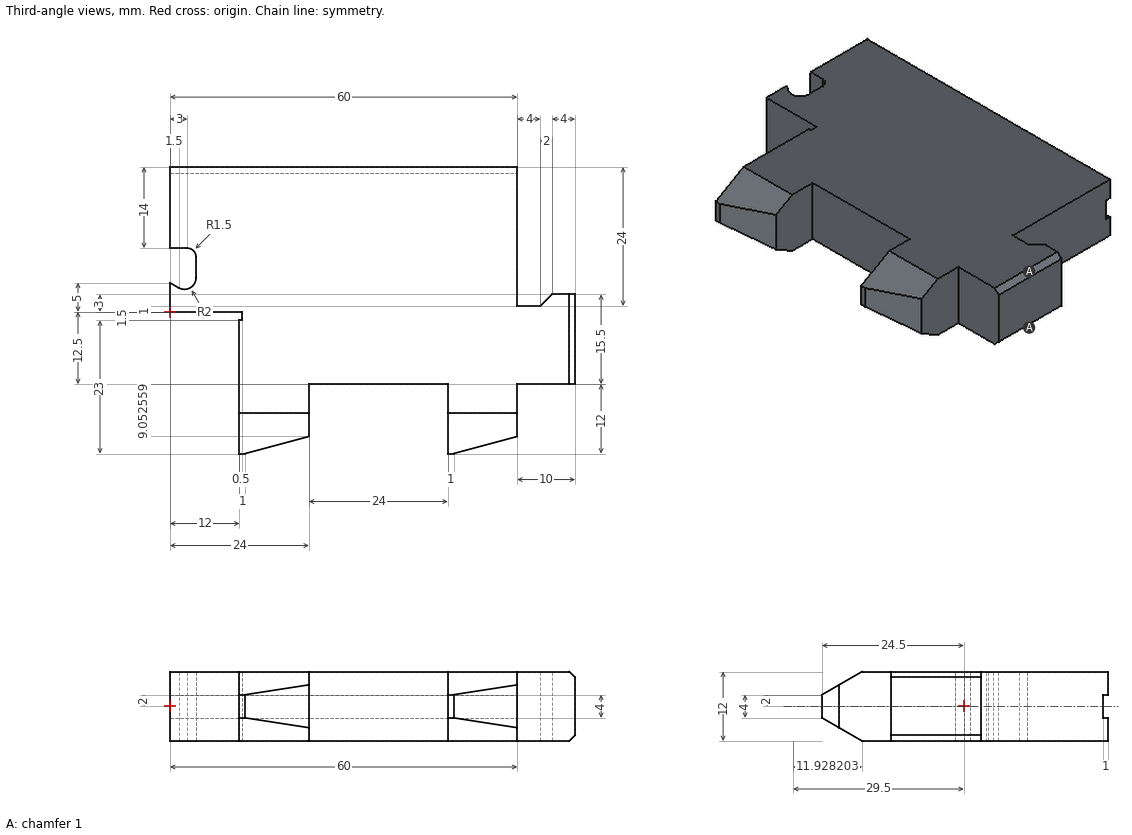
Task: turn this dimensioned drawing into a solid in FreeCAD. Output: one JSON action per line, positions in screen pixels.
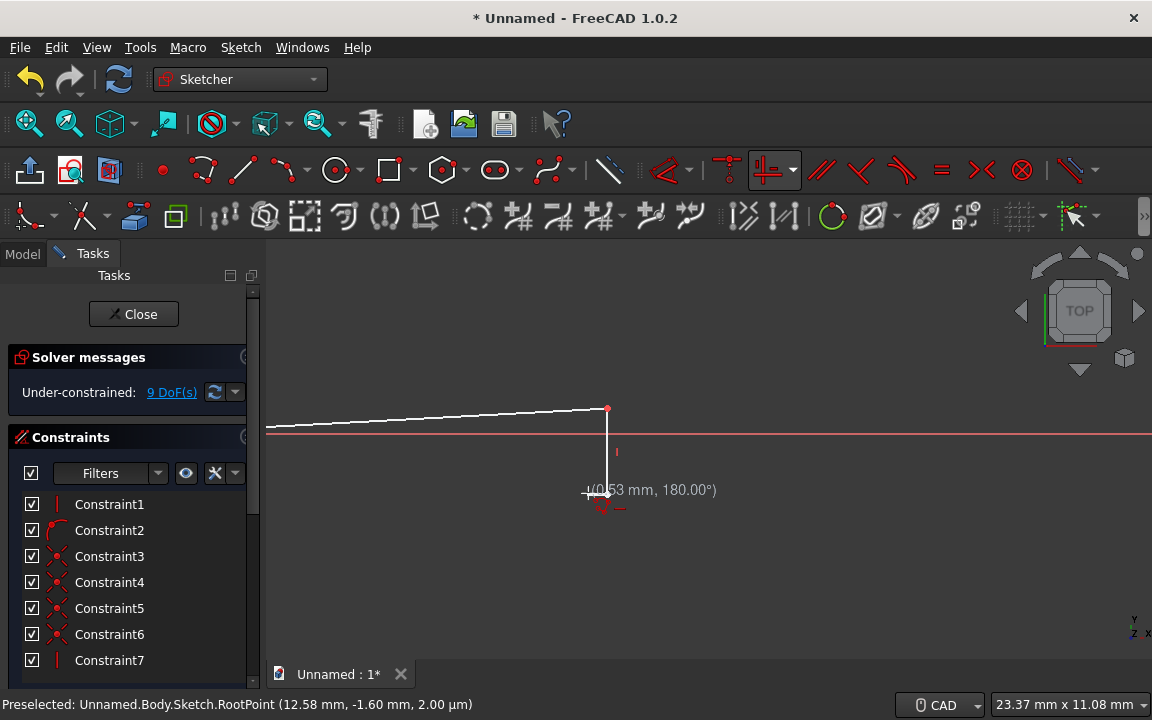
{"action": "left_click", "coordinate": [588, 492]}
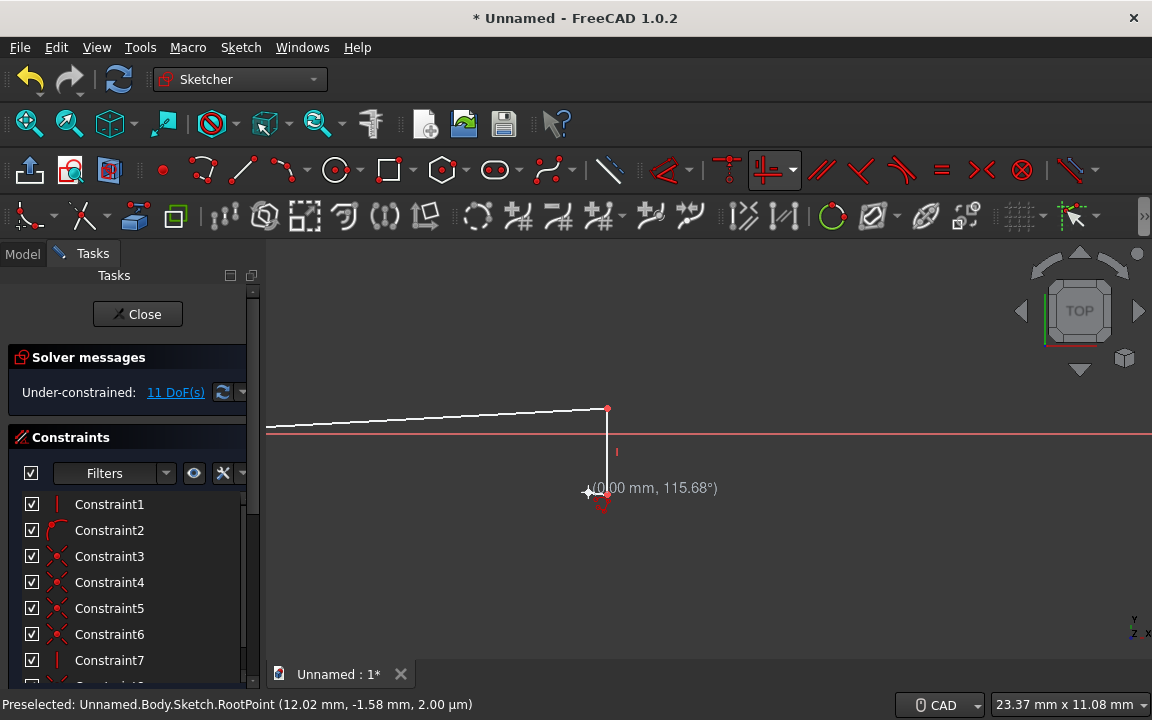
{"action": "scroll", "coordinate": [512, 453], "scroll_direction": "down", "scroll_amount": 10}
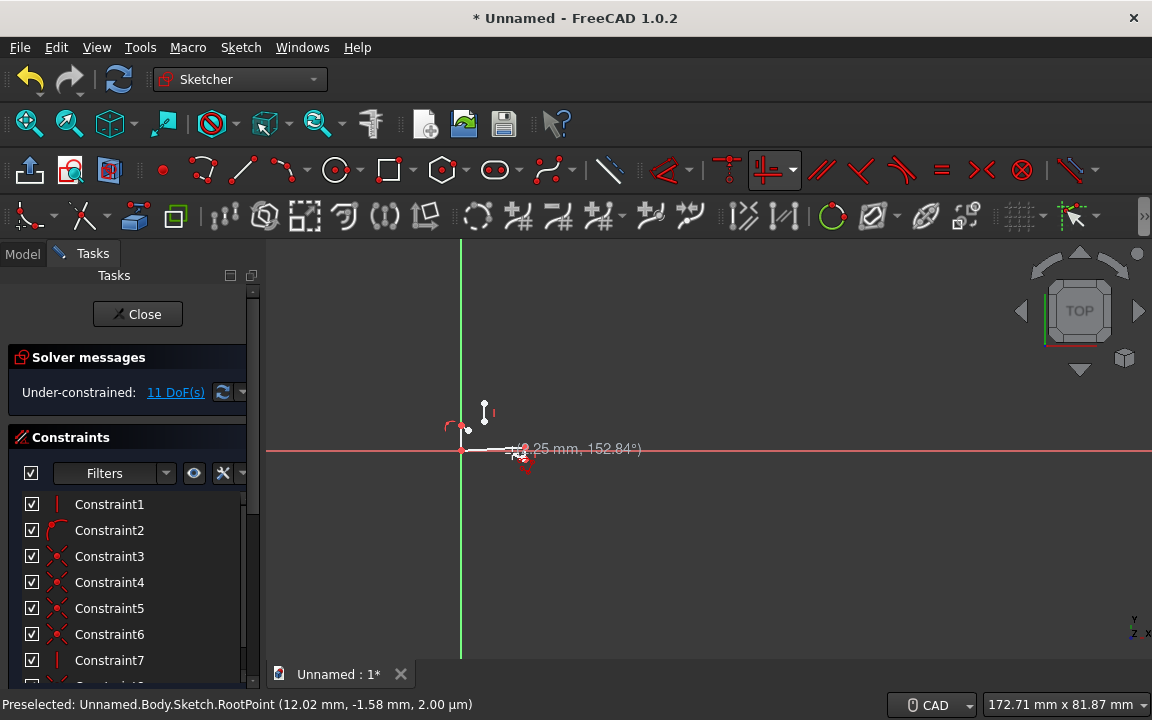
{"action": "left_click", "coordinate": [523, 577]}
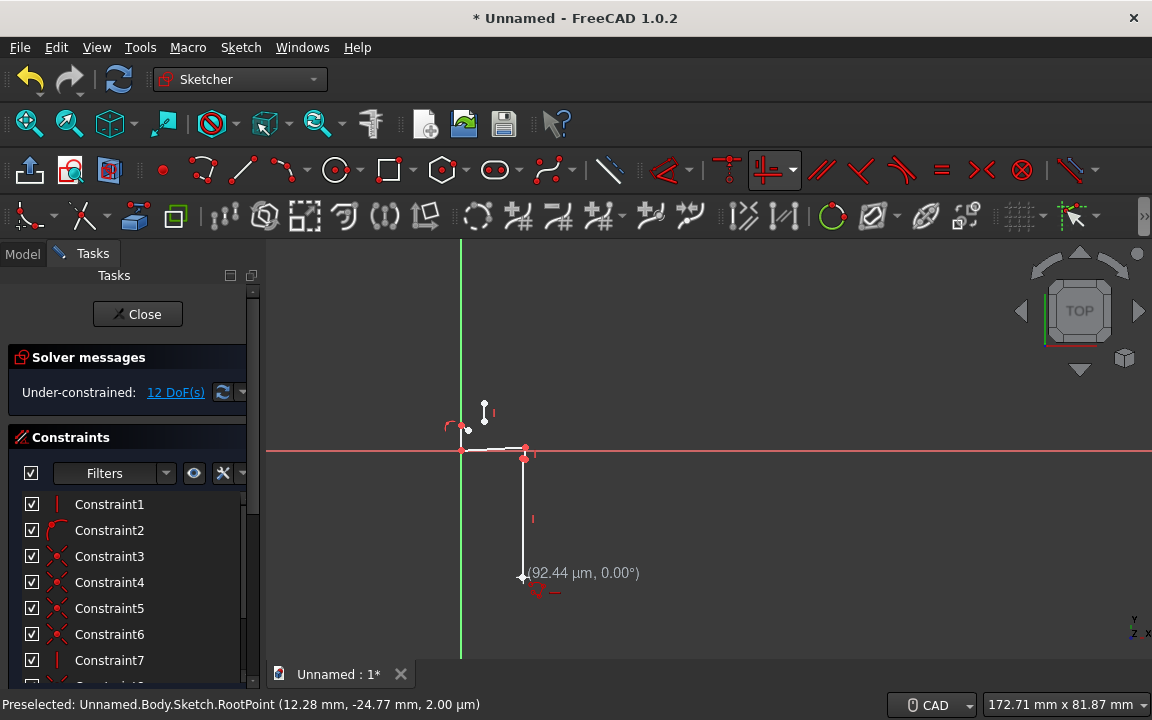
{"action": "scroll", "coordinate": [528, 577], "scroll_direction": "up", "scroll_amount": 6}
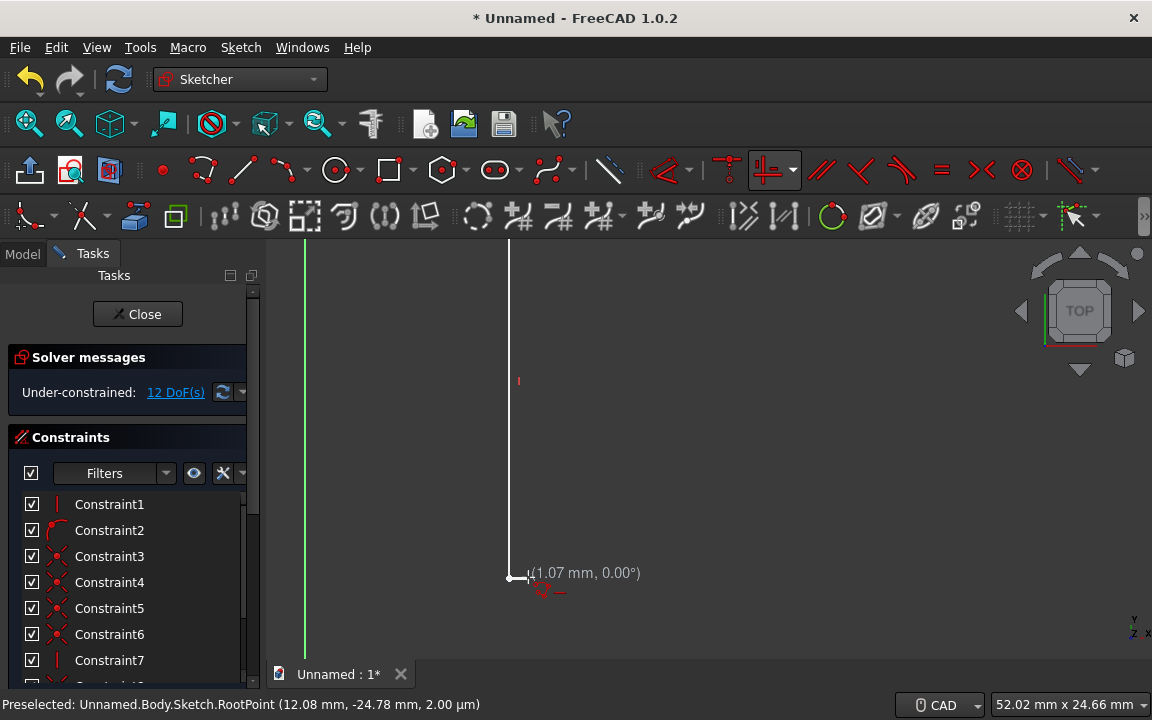
{"action": "left_click", "coordinate": [526, 575]}
{"action": "left_click", "coordinate": [714, 524]}
{"action": "left_click", "coordinate": [714, 369]}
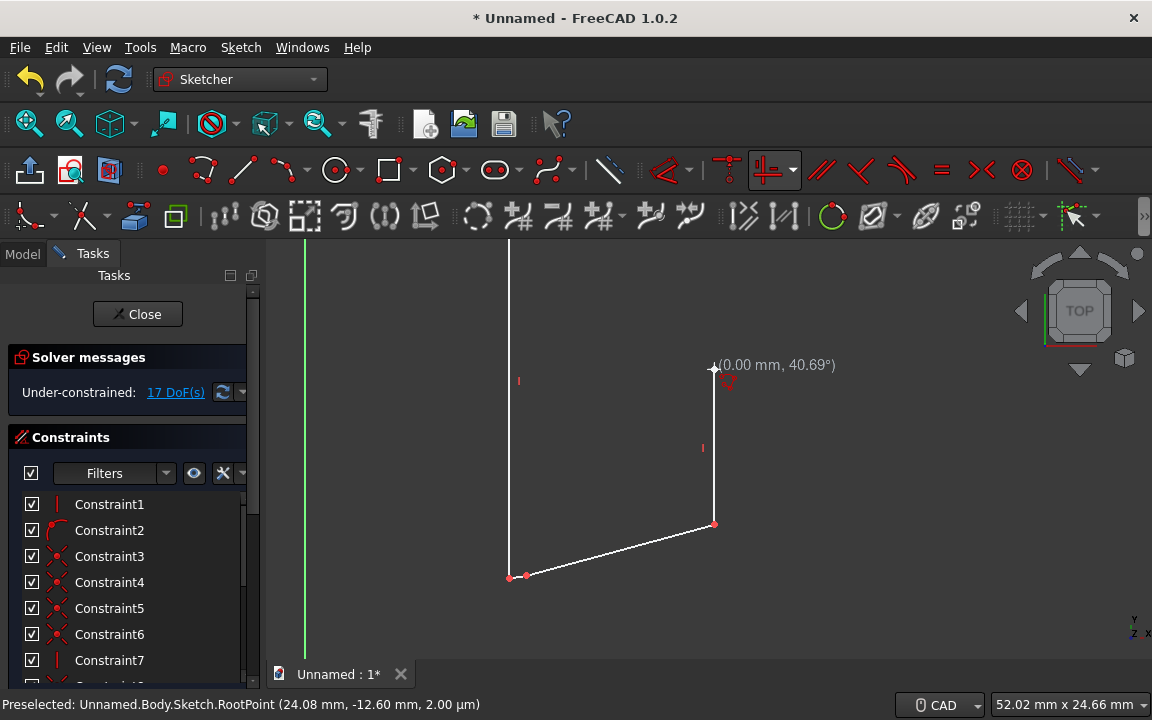
{"action": "scroll", "coordinate": [528, 577], "scroll_direction": "down", "scroll_amount": 6}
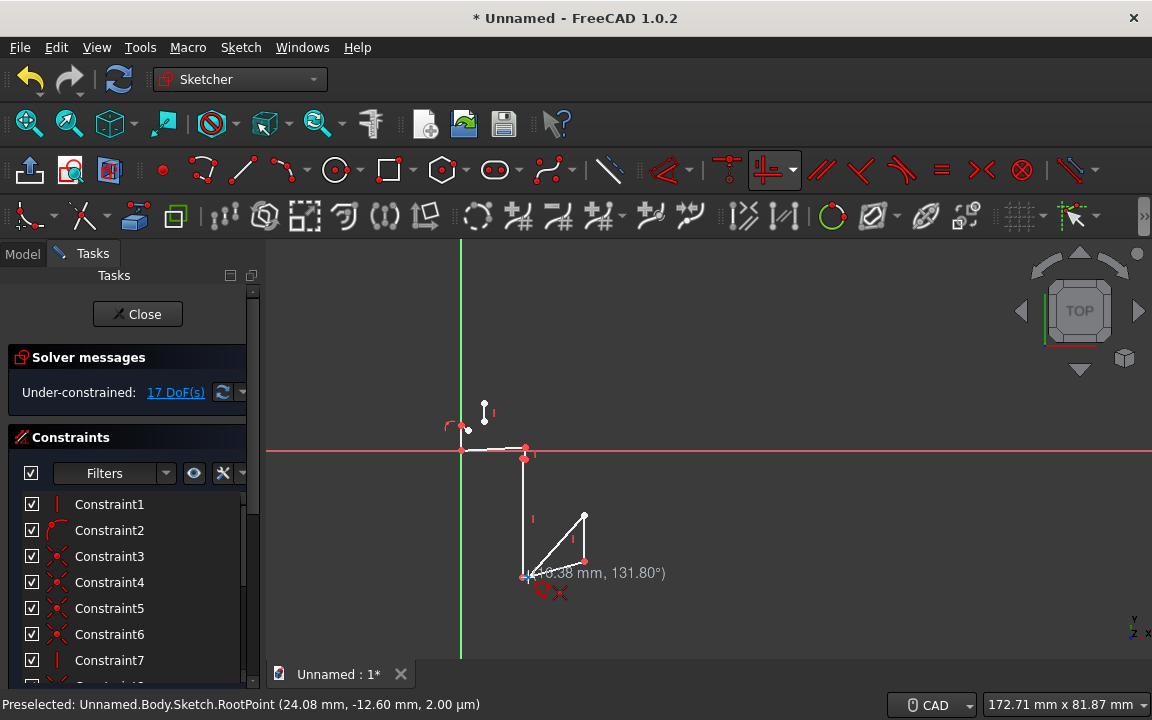
{"action": "left_click", "coordinate": [707, 515]}
{"action": "left_click", "coordinate": [707, 577]}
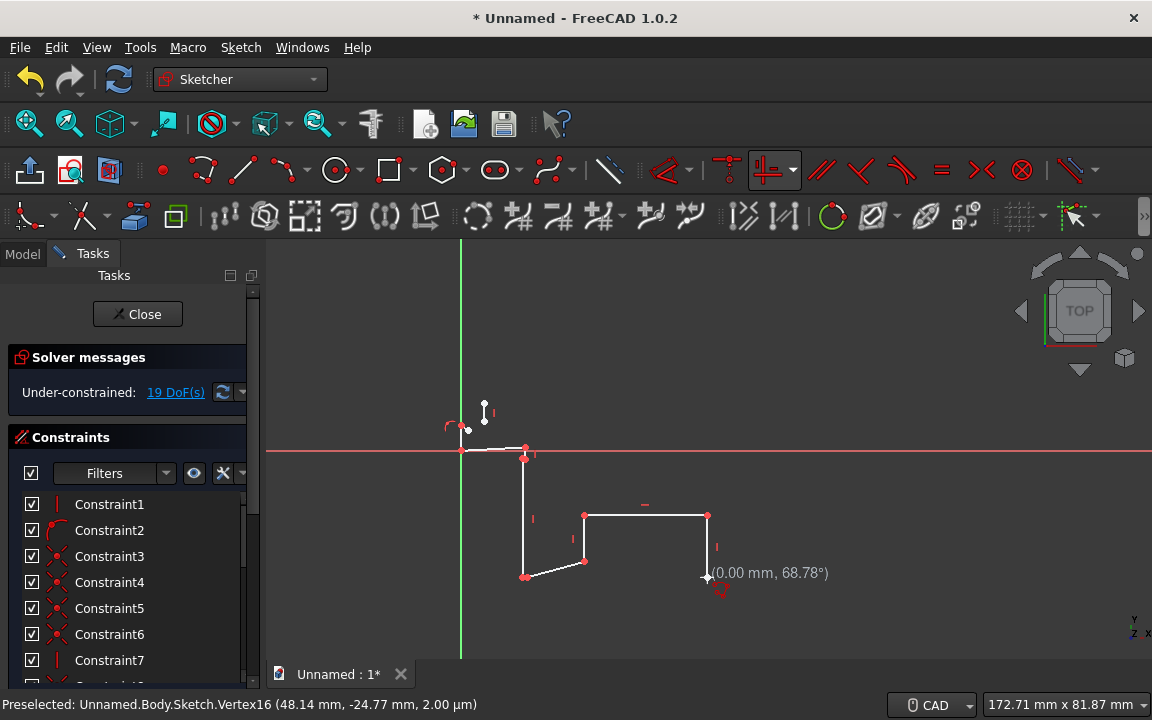
{"action": "scroll", "coordinate": [712, 577], "scroll_direction": "up", "scroll_amount": 6}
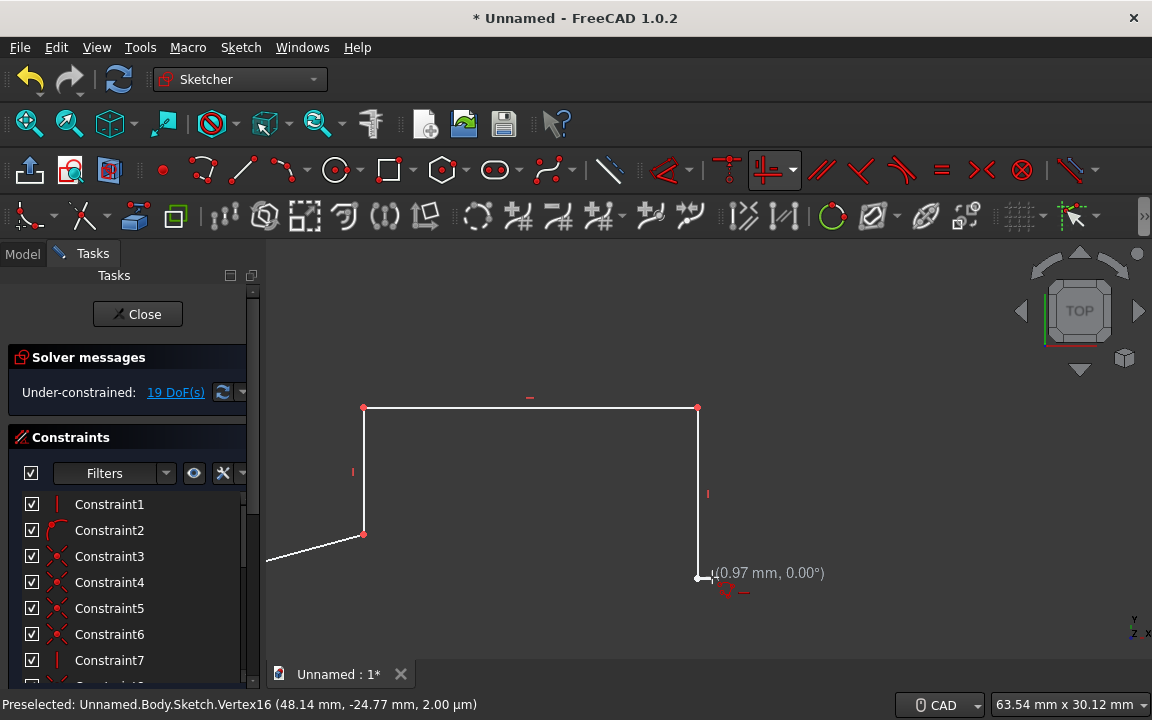
{"action": "left_click", "coordinate": [712, 575]}
{"action": "left_click", "coordinate": [899, 524]}
{"action": "left_click", "coordinate": [899, 369]}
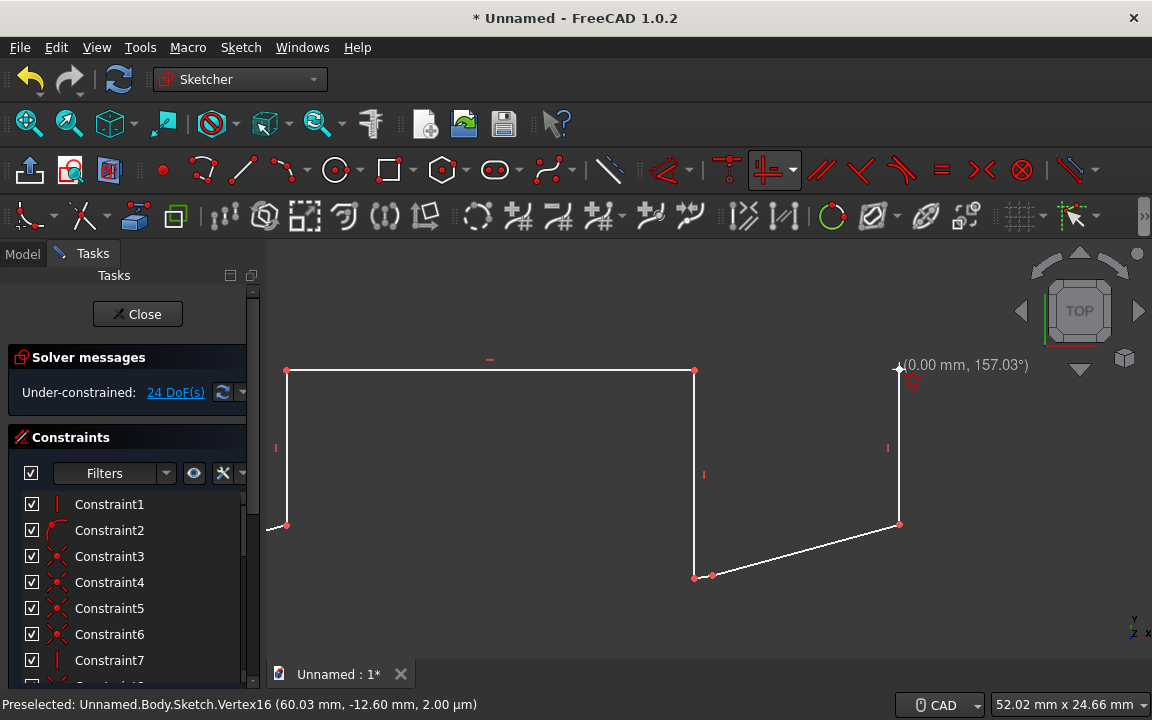
{"action": "scroll", "coordinate": [712, 577], "scroll_direction": "down", "scroll_amount": 6}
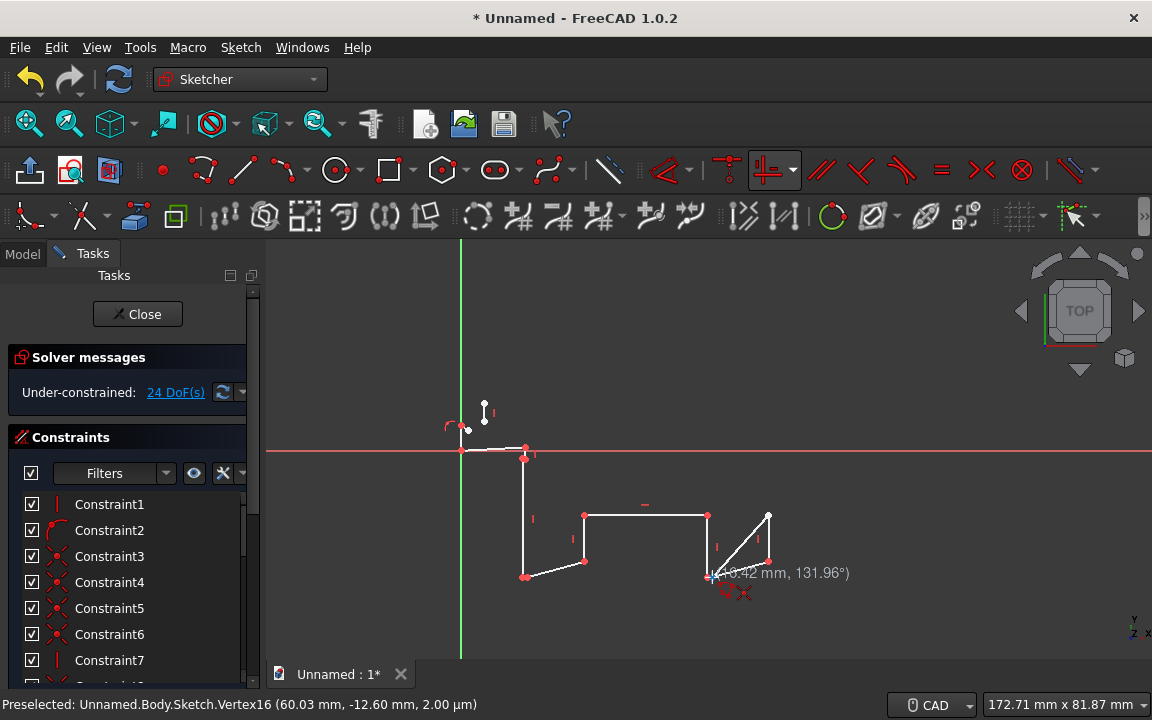
{"action": "left_click", "coordinate": [820, 515]}
{"action": "left_click", "coordinate": [820, 436]}
{"action": "left_click", "coordinate": [800, 436]}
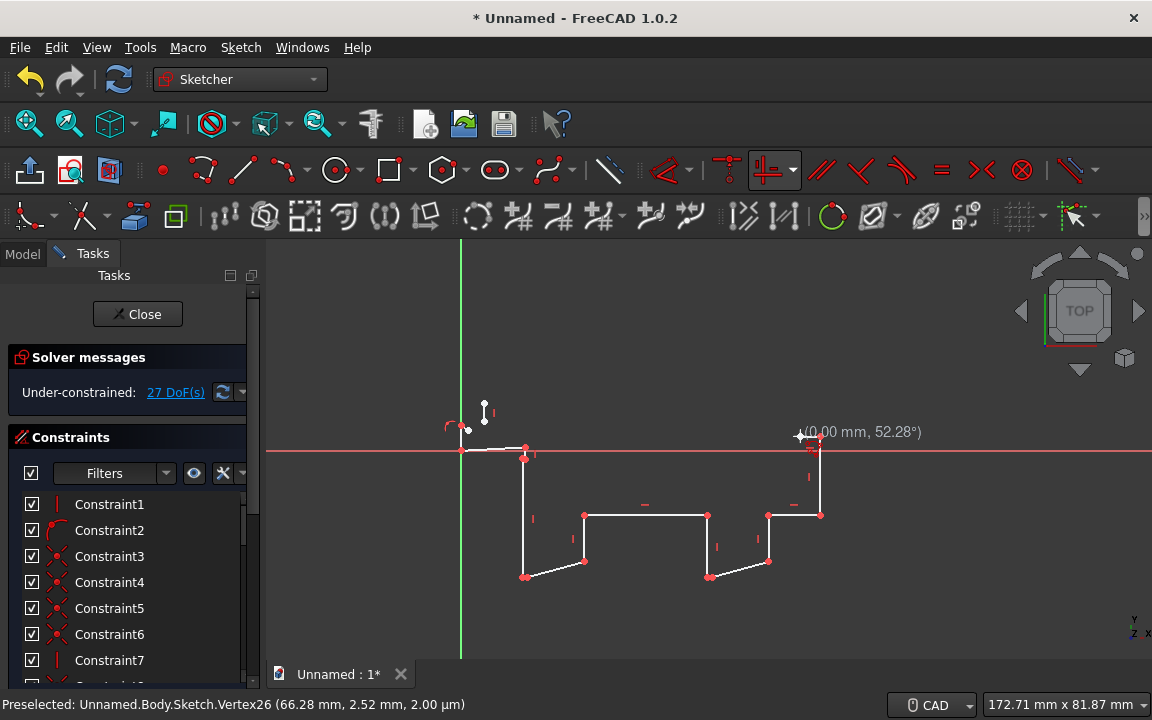
{"action": "scroll", "coordinate": [789, 446], "scroll_direction": "up", "scroll_amount": 6}